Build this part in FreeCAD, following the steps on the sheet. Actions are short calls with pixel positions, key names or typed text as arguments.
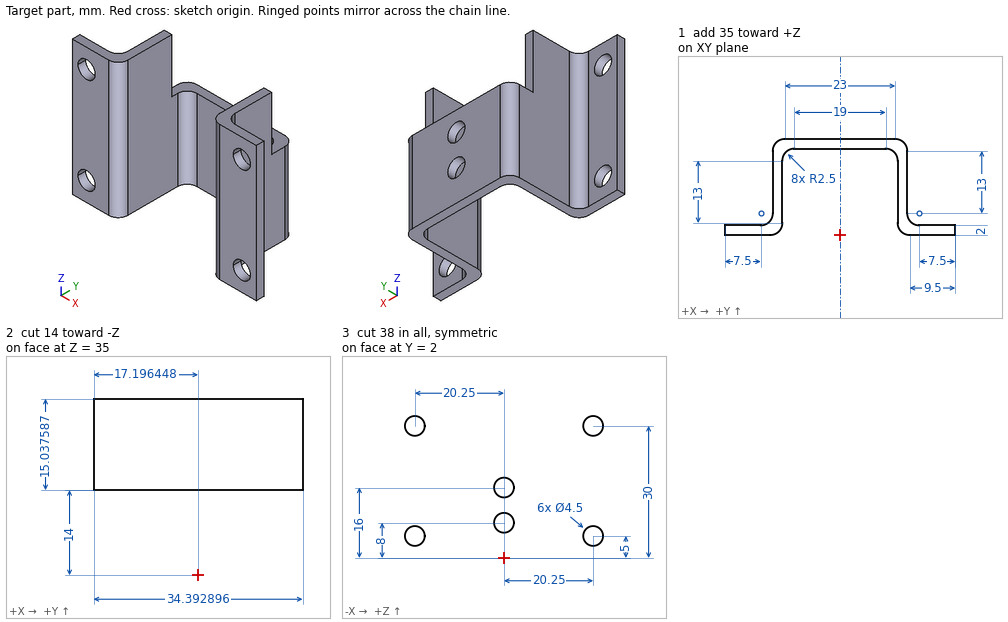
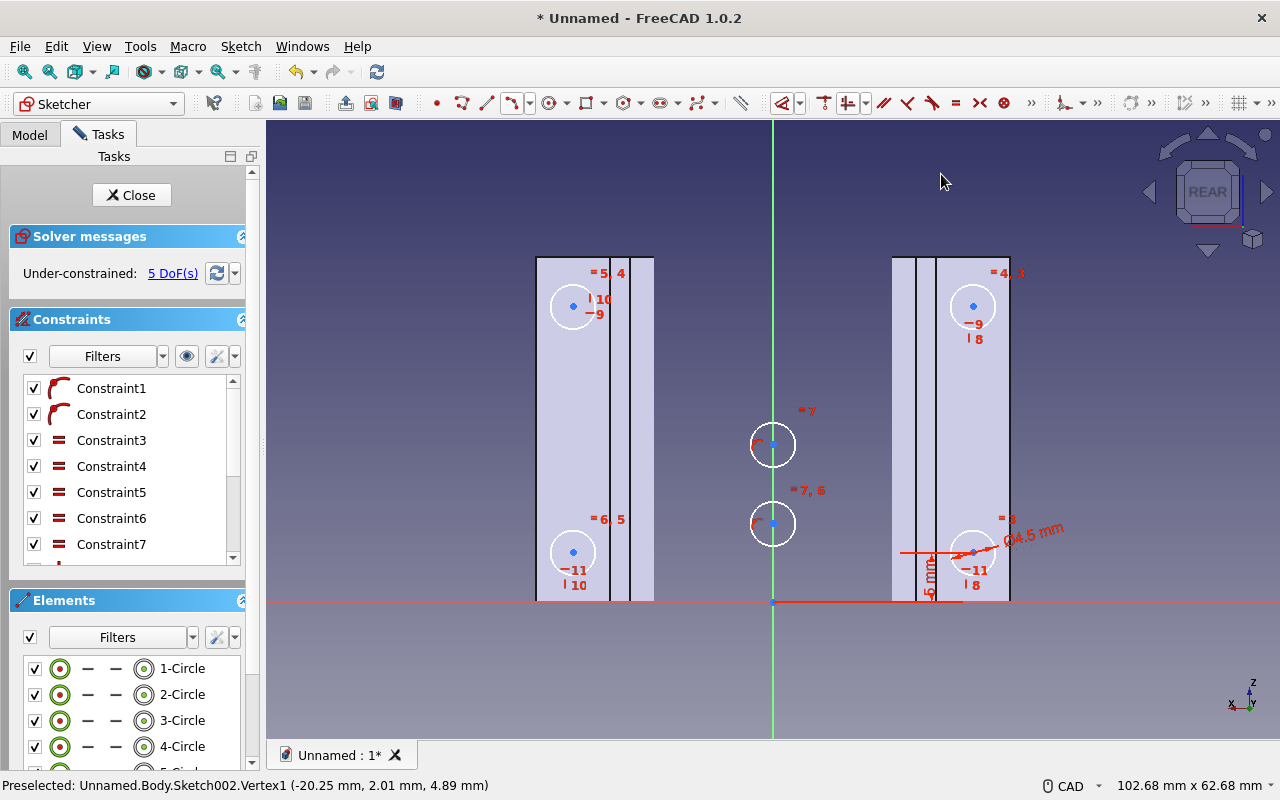
click(773, 524)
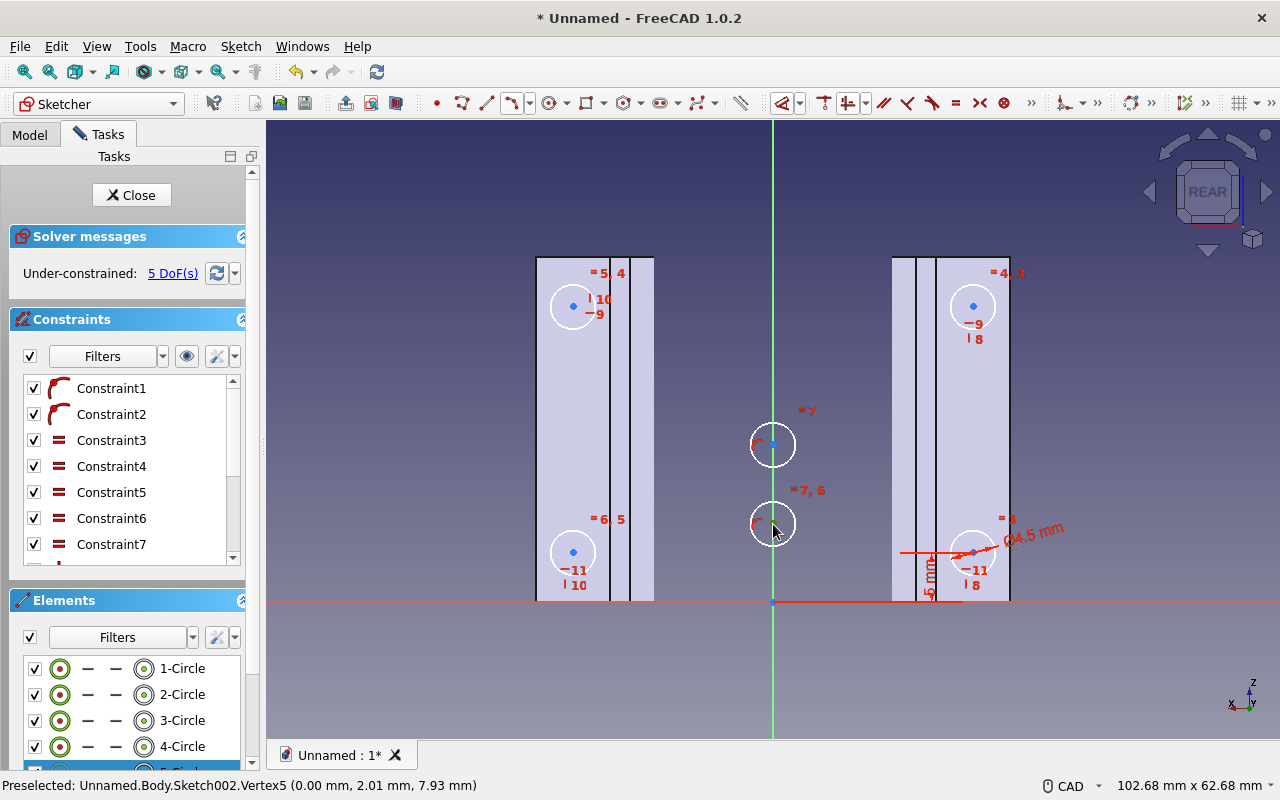
key(i)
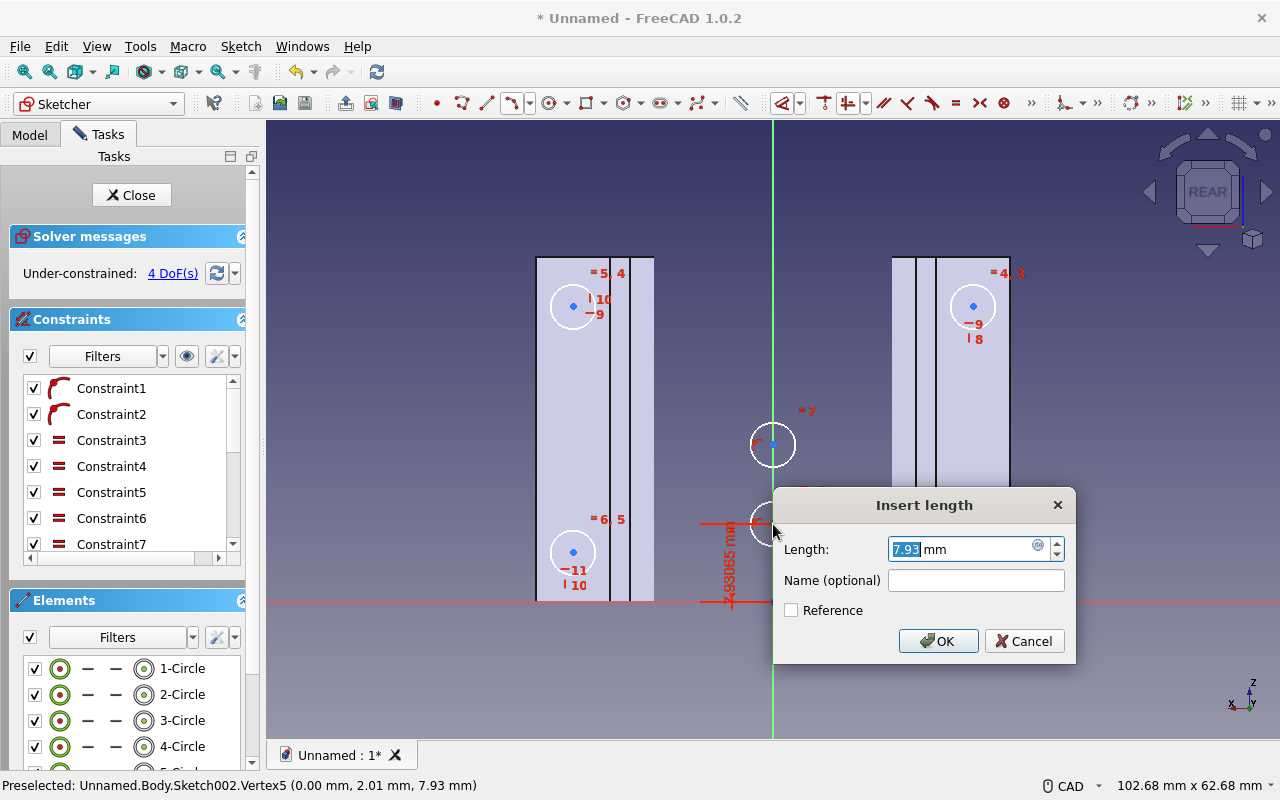
text(8)
key(Return)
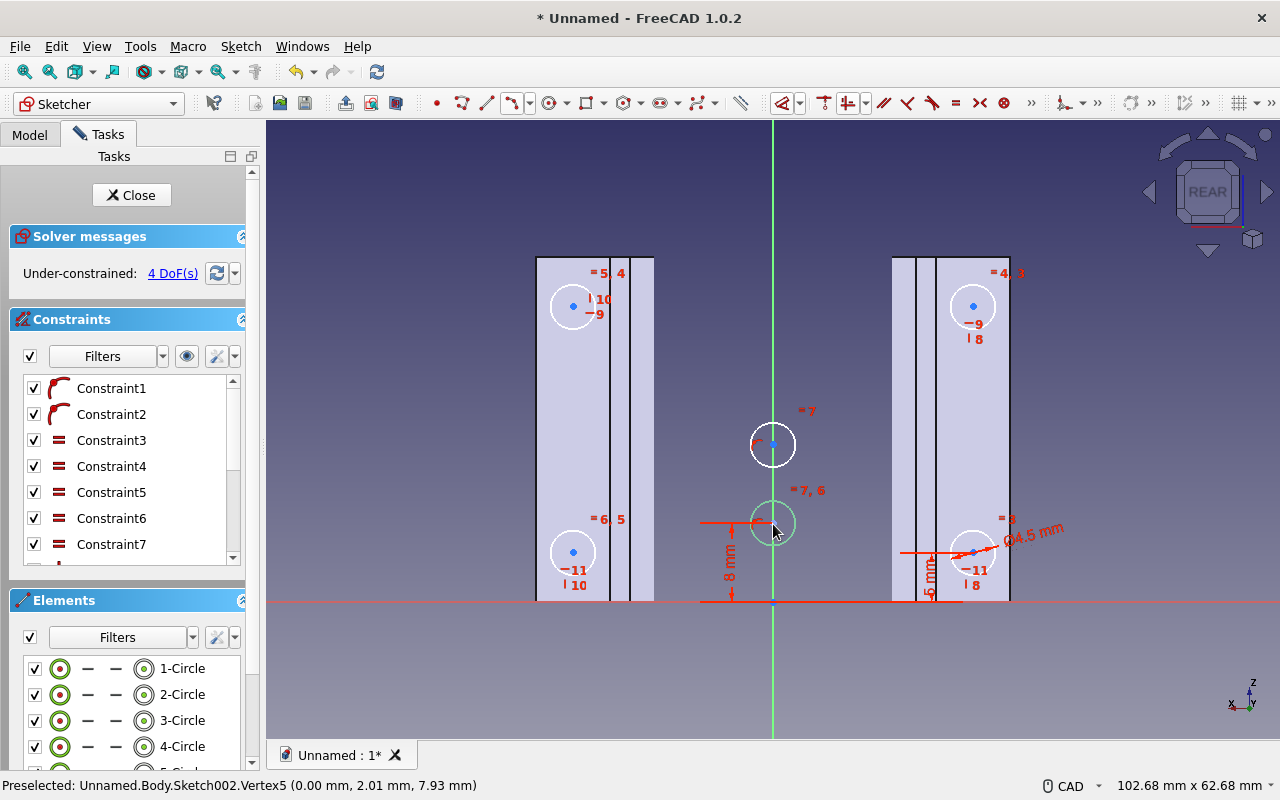
click(973, 307)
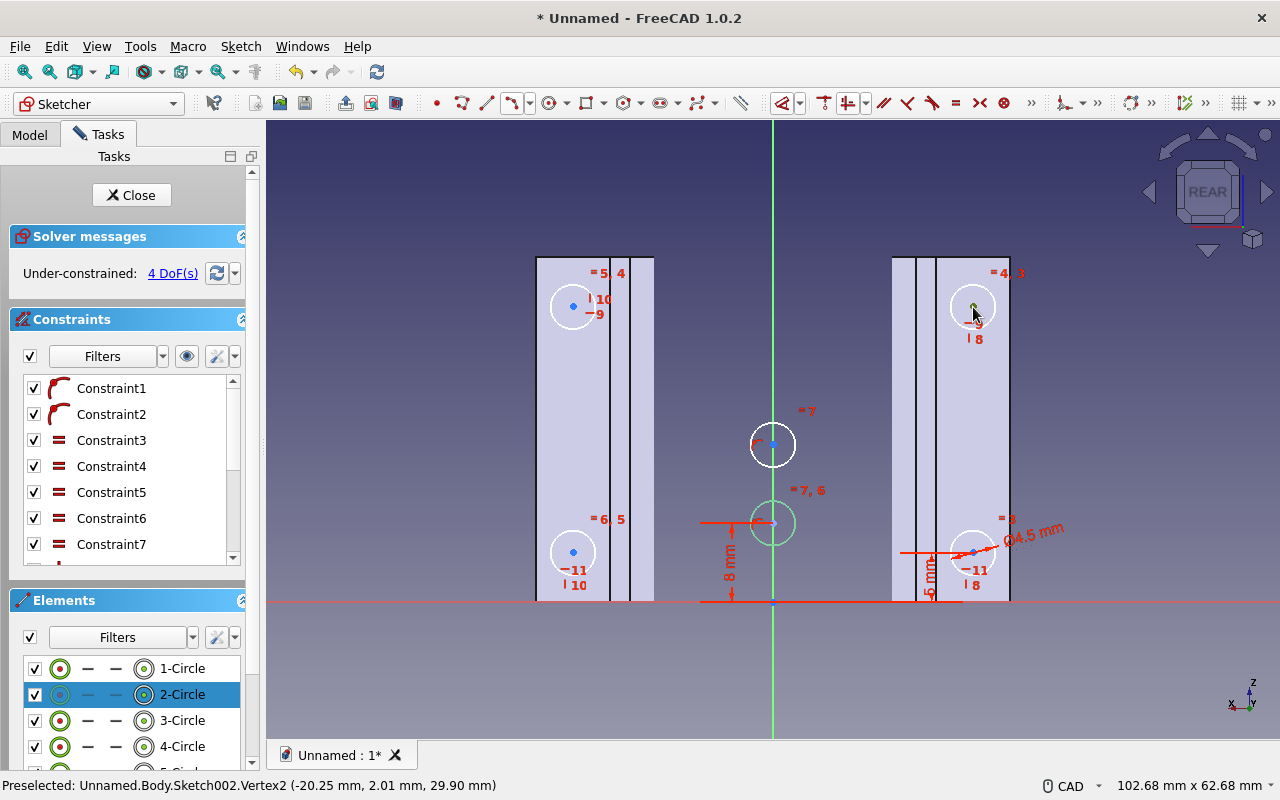
key(i)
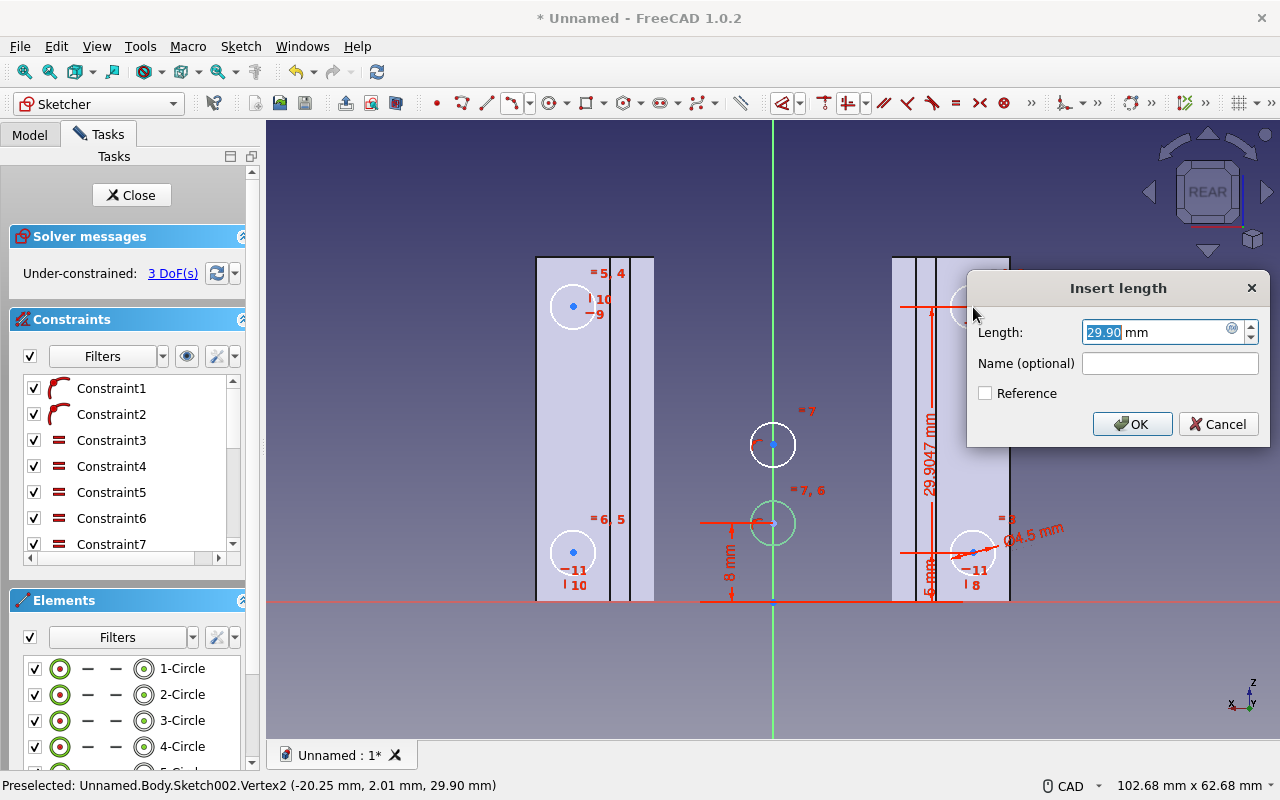
text(30)
key(Return)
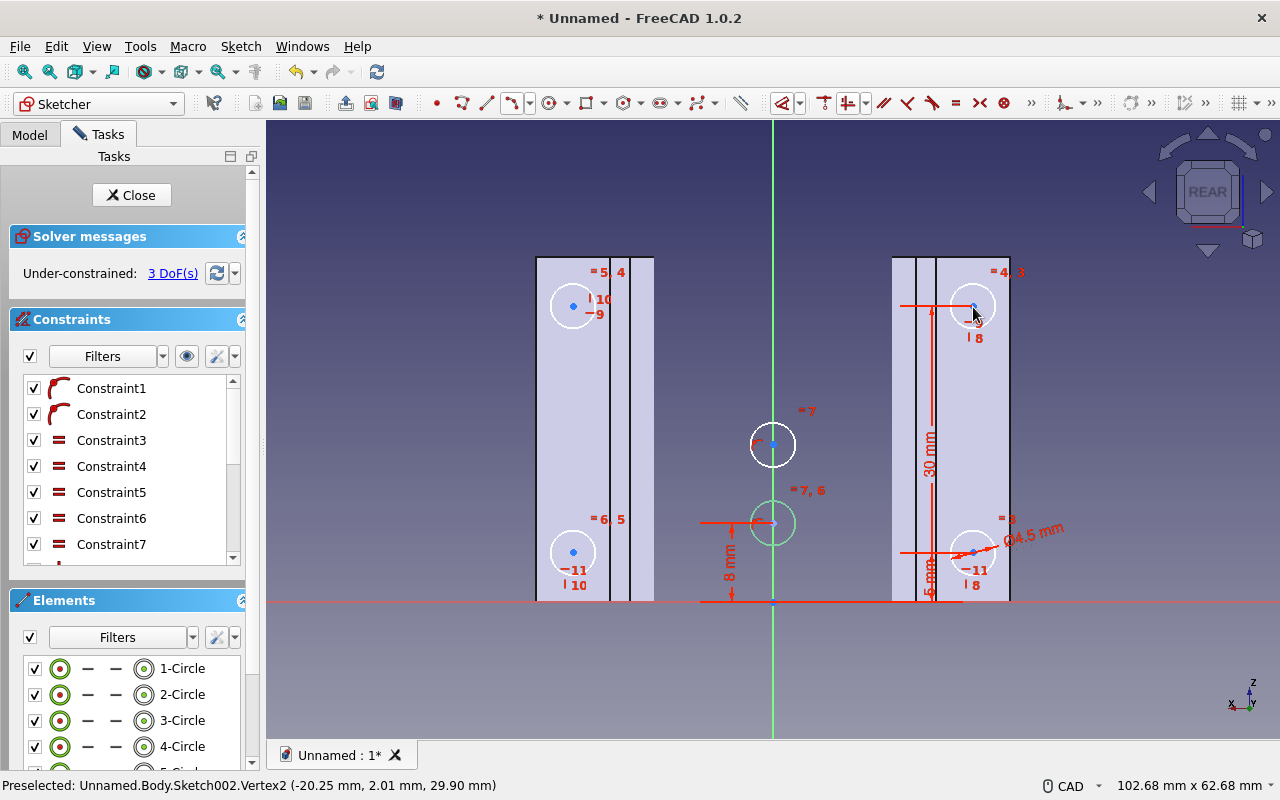
click(773, 445)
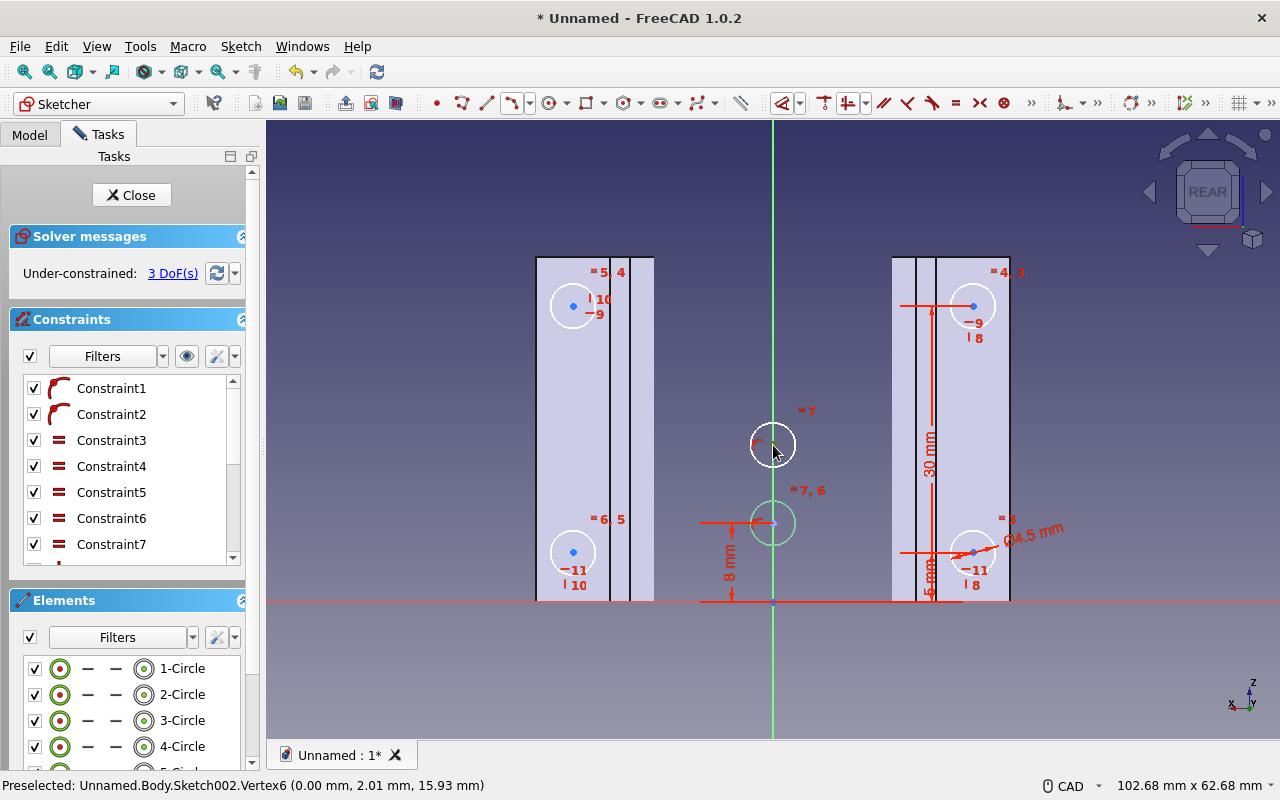
key(i)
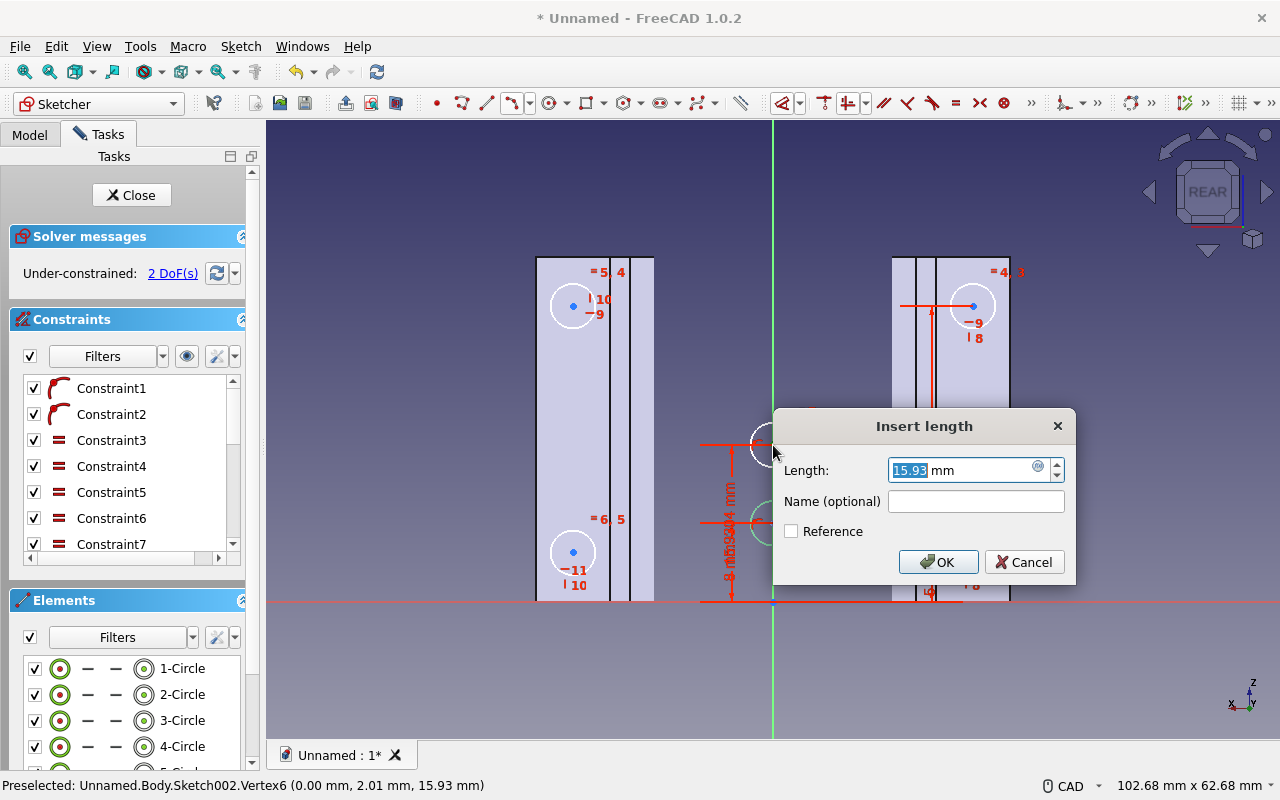
text(16)
key(Return)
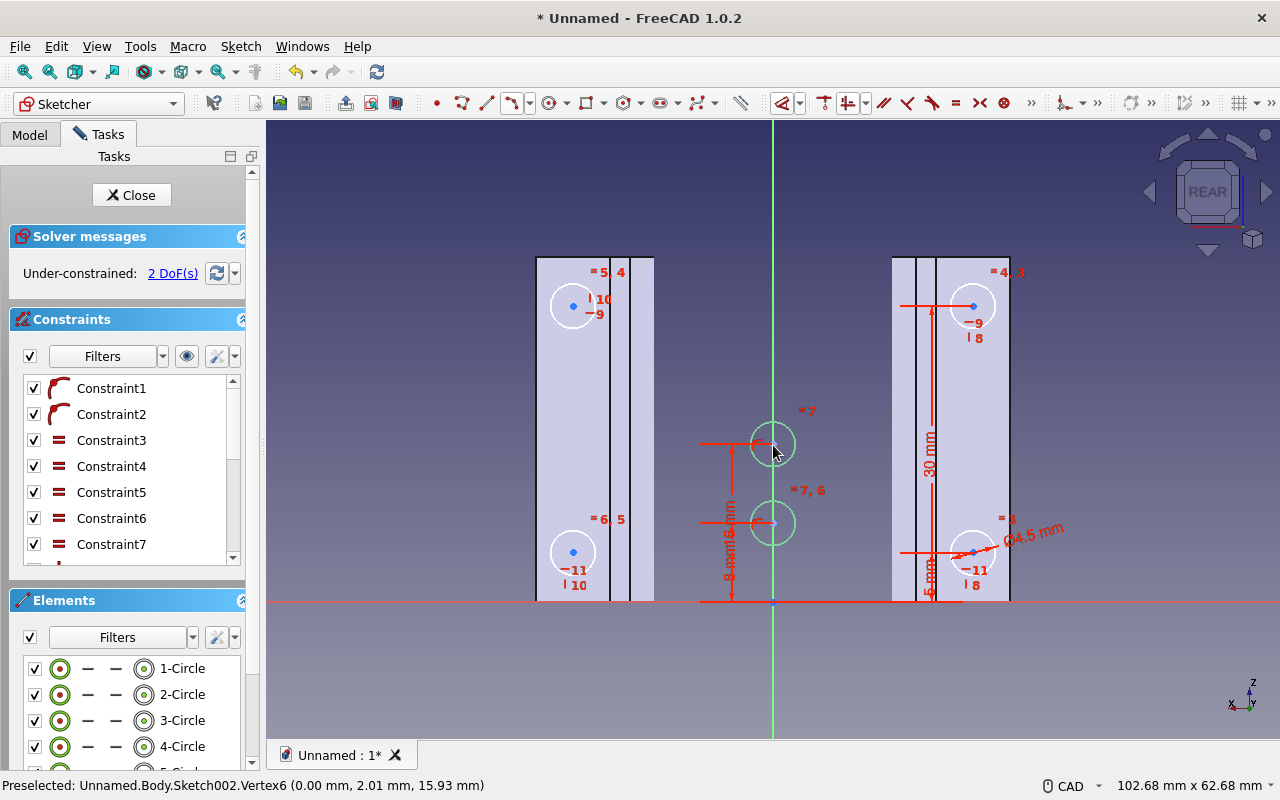
click(973, 553)